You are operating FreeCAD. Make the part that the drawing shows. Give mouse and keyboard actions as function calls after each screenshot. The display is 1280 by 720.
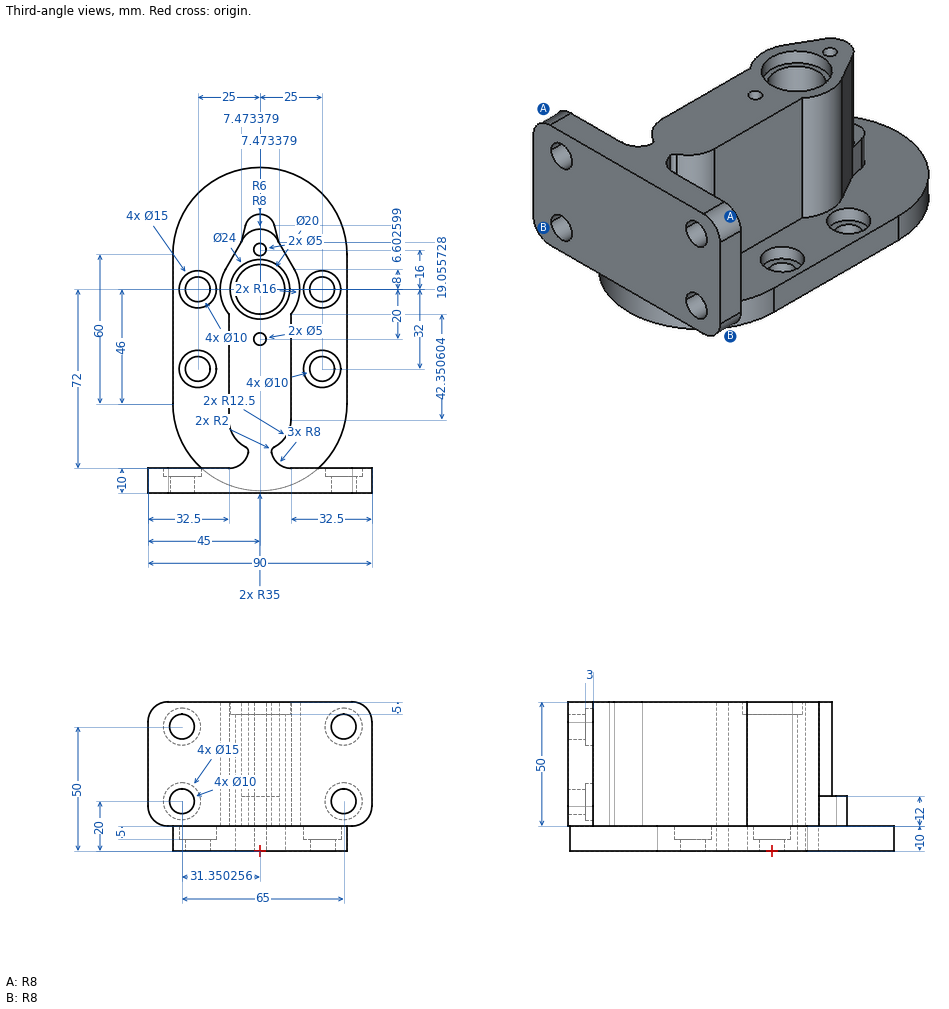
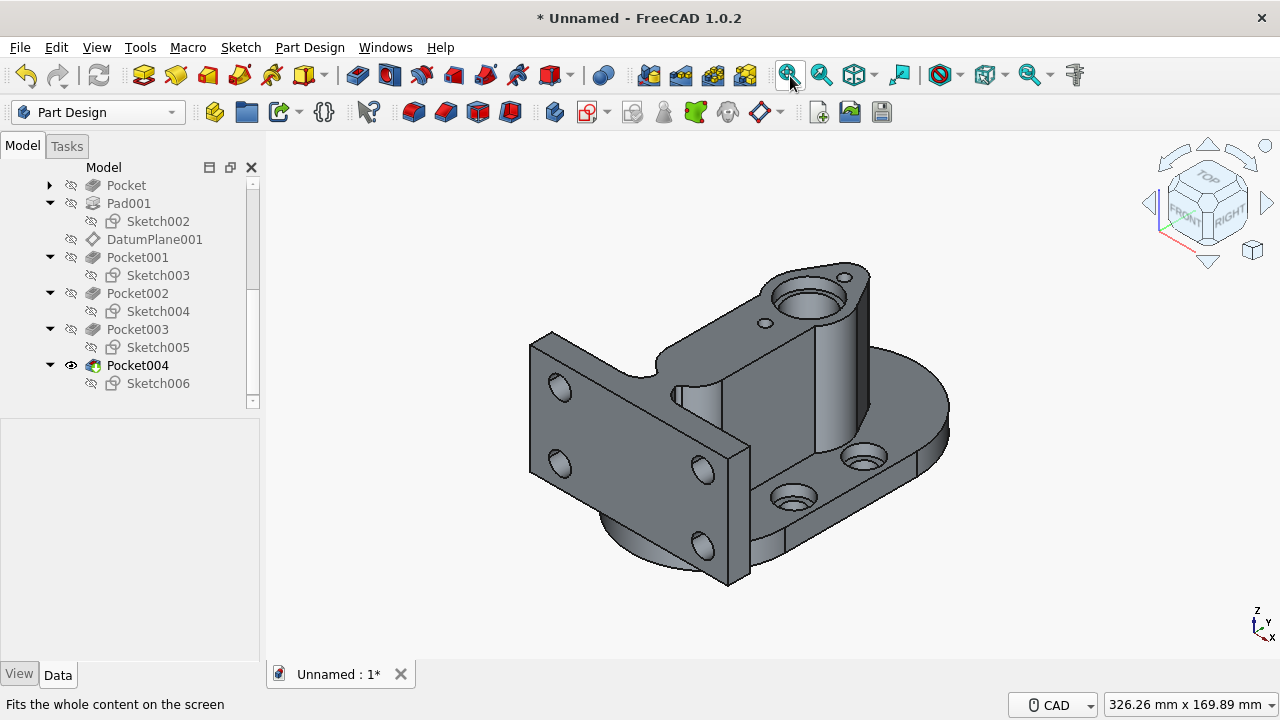
click(904, 420)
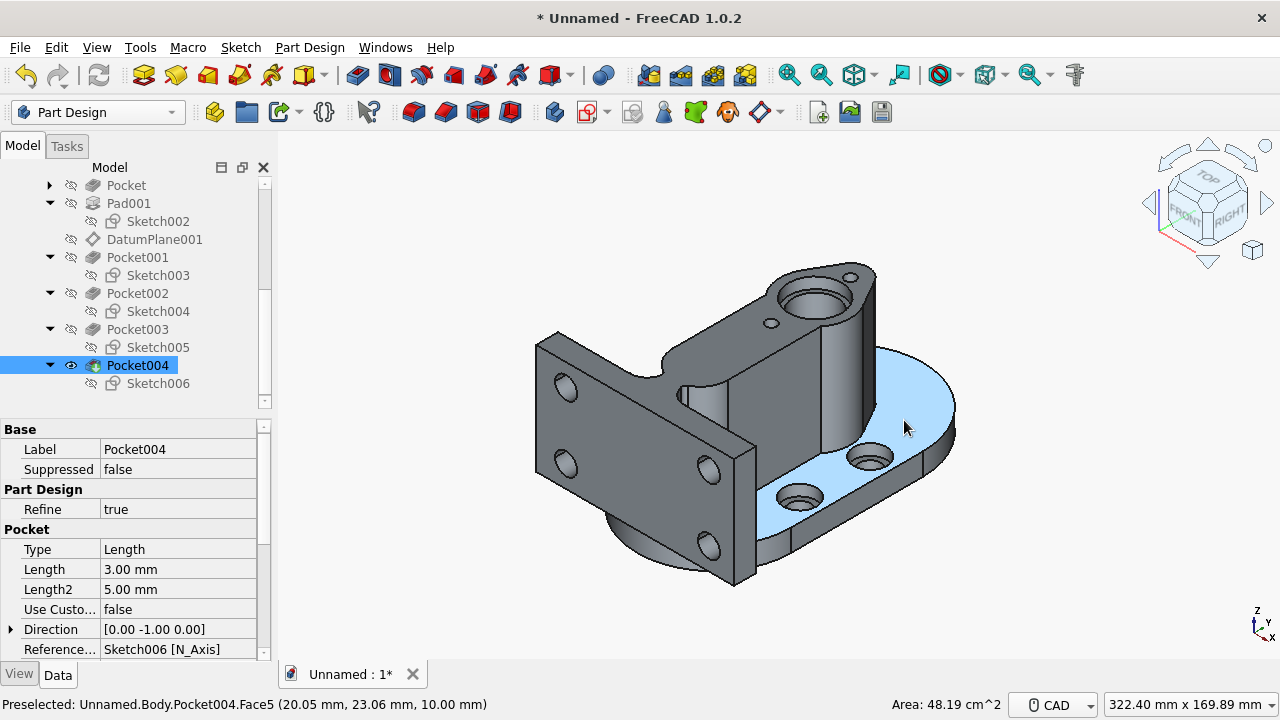
click(588, 112)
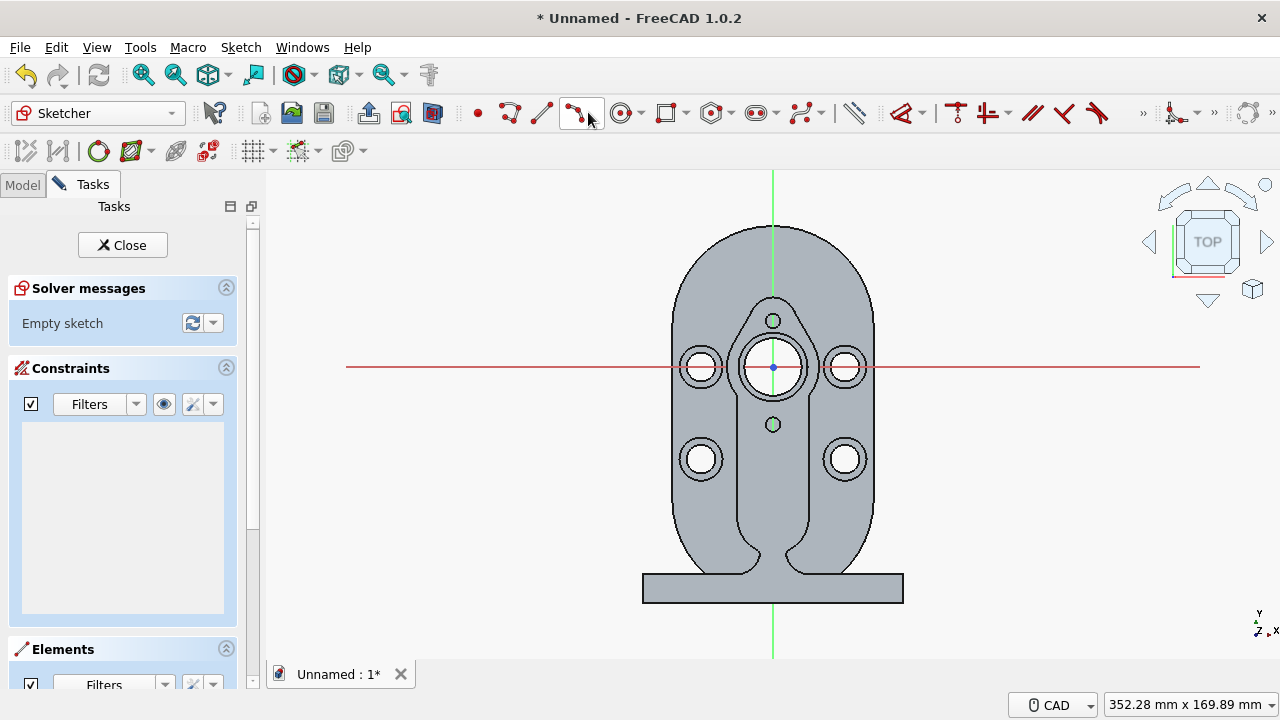
click(434, 114)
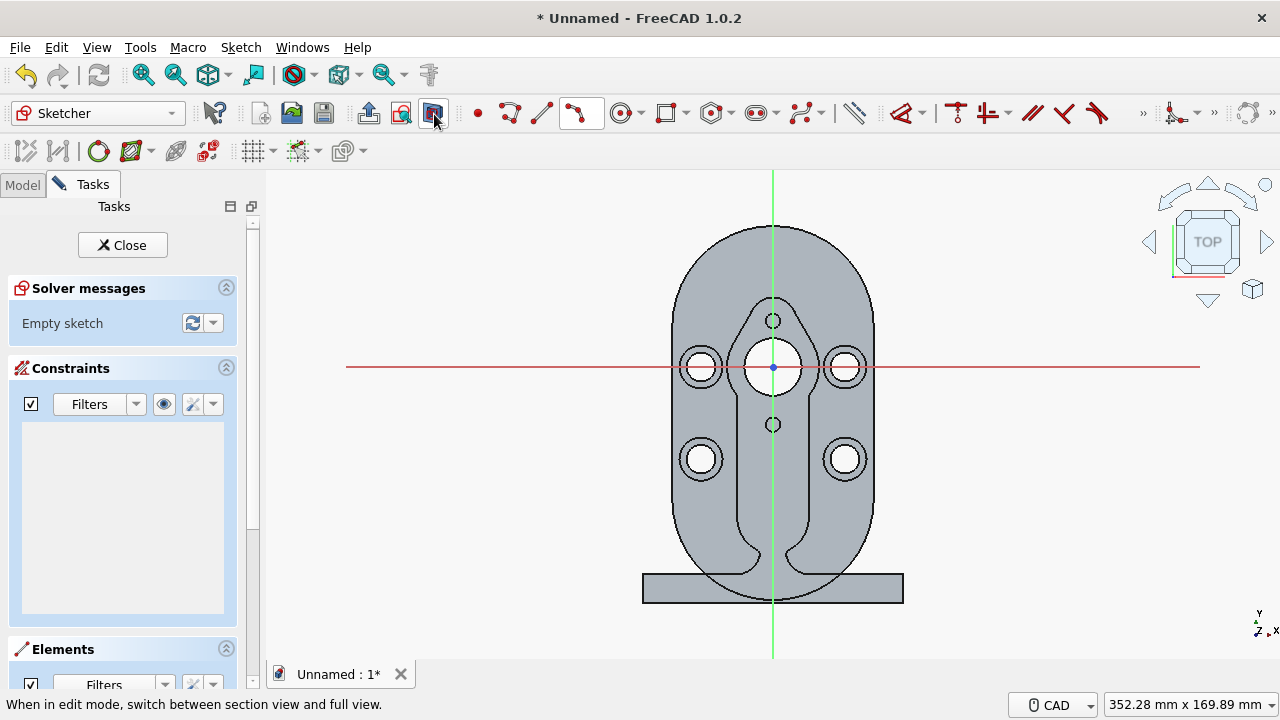
scroll(803, 284, up, 6)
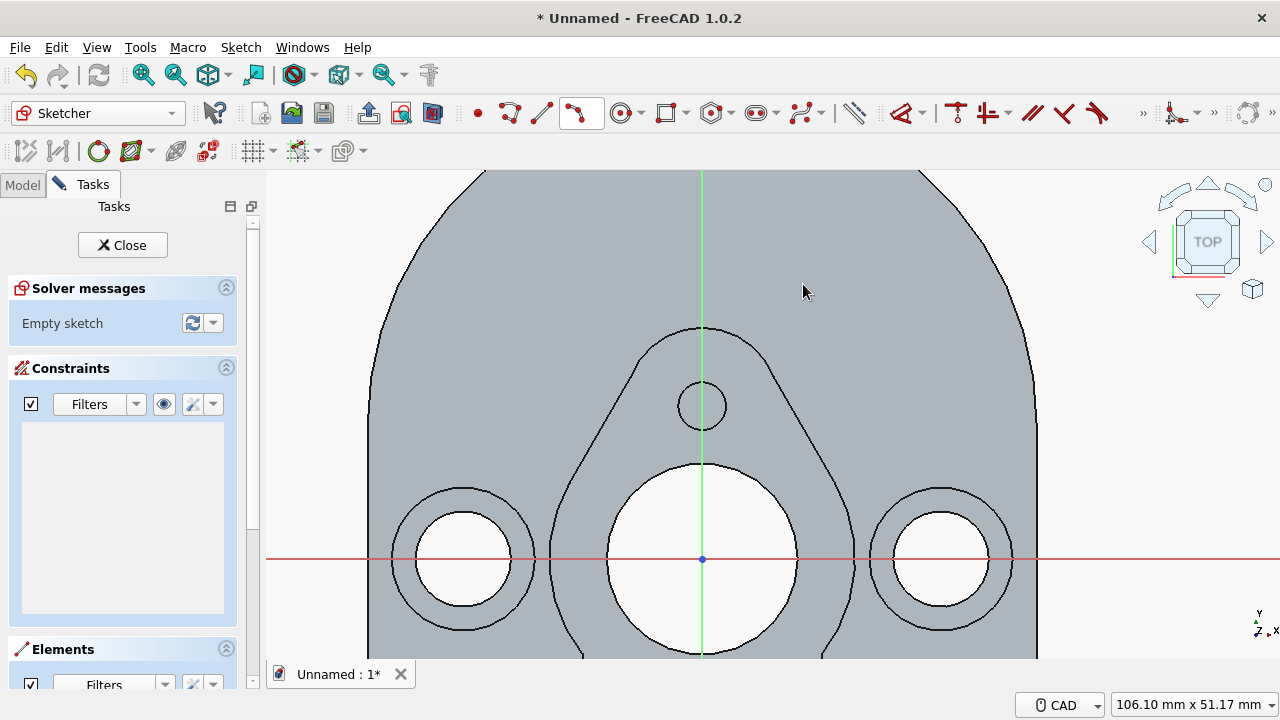
click(542, 114)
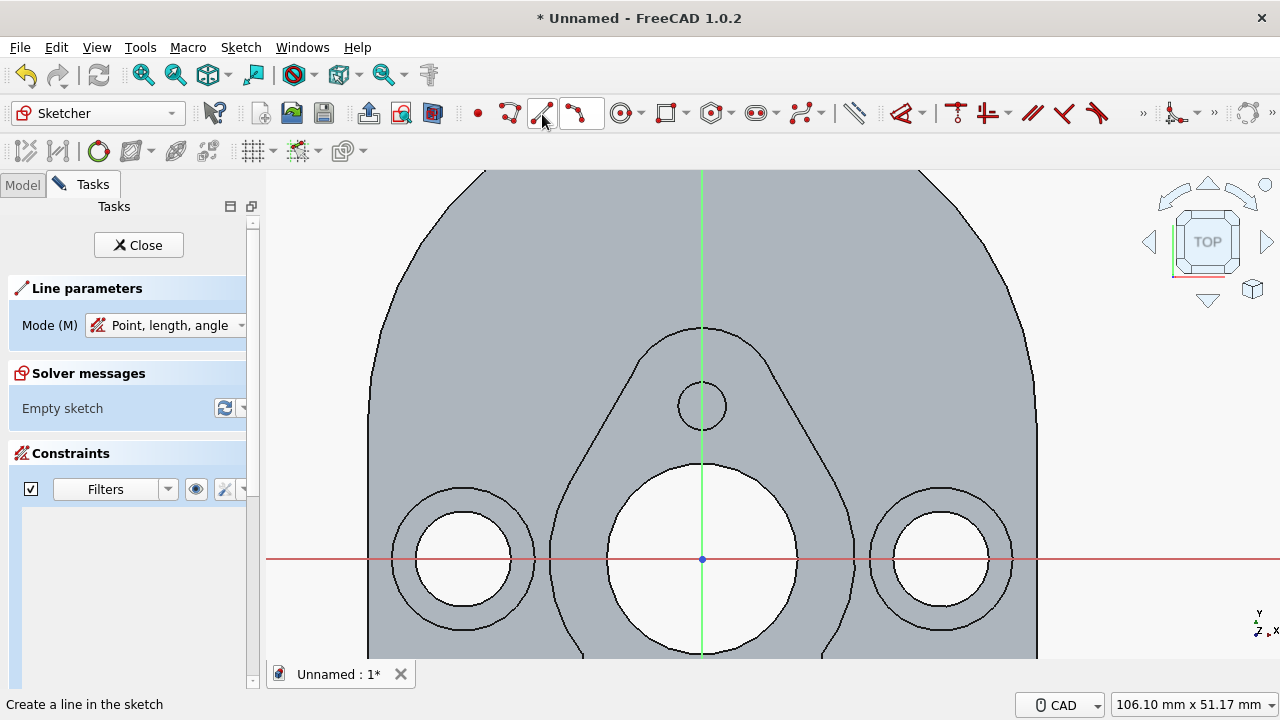
click(774, 377)
click(758, 314)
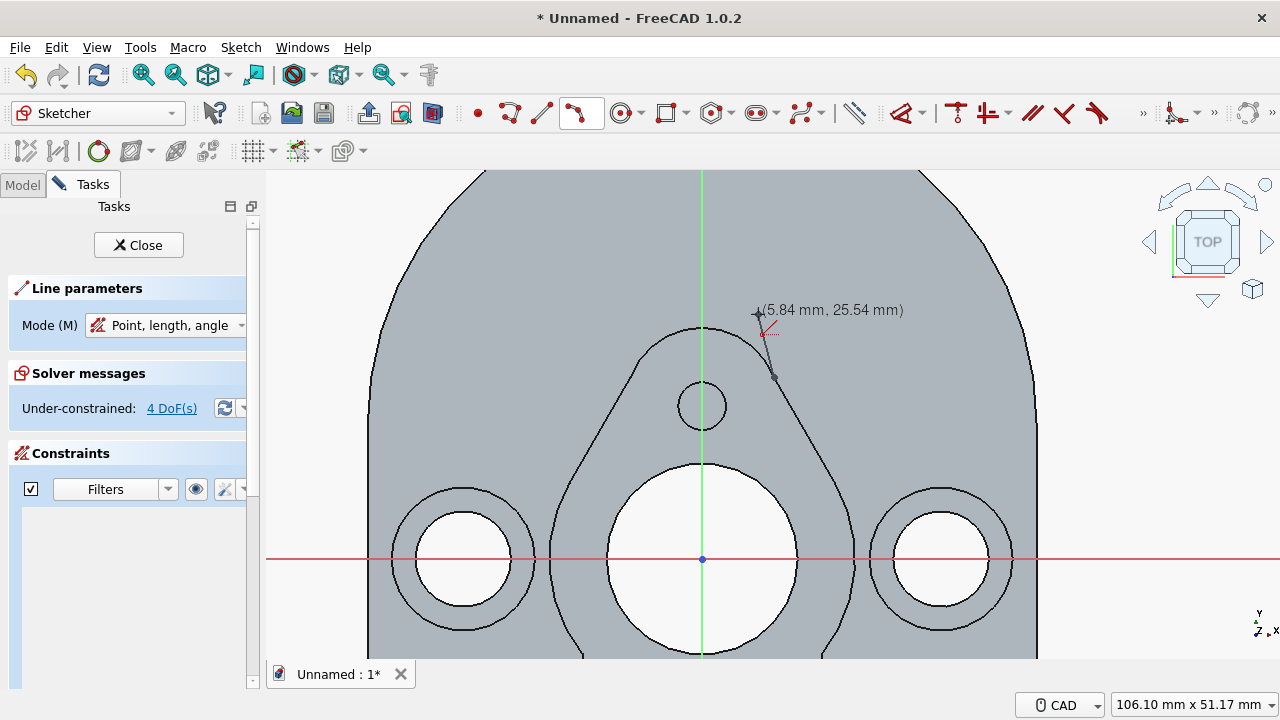
click(647, 314)
click(631, 377)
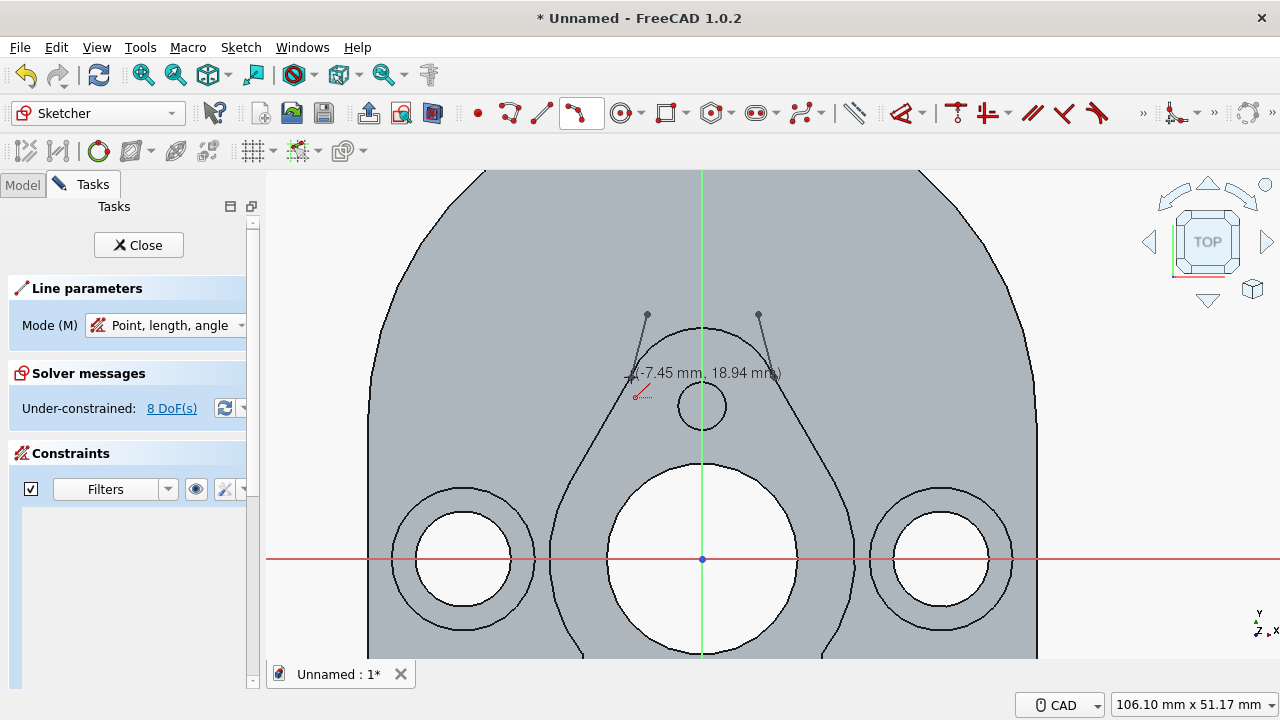
click(576, 114)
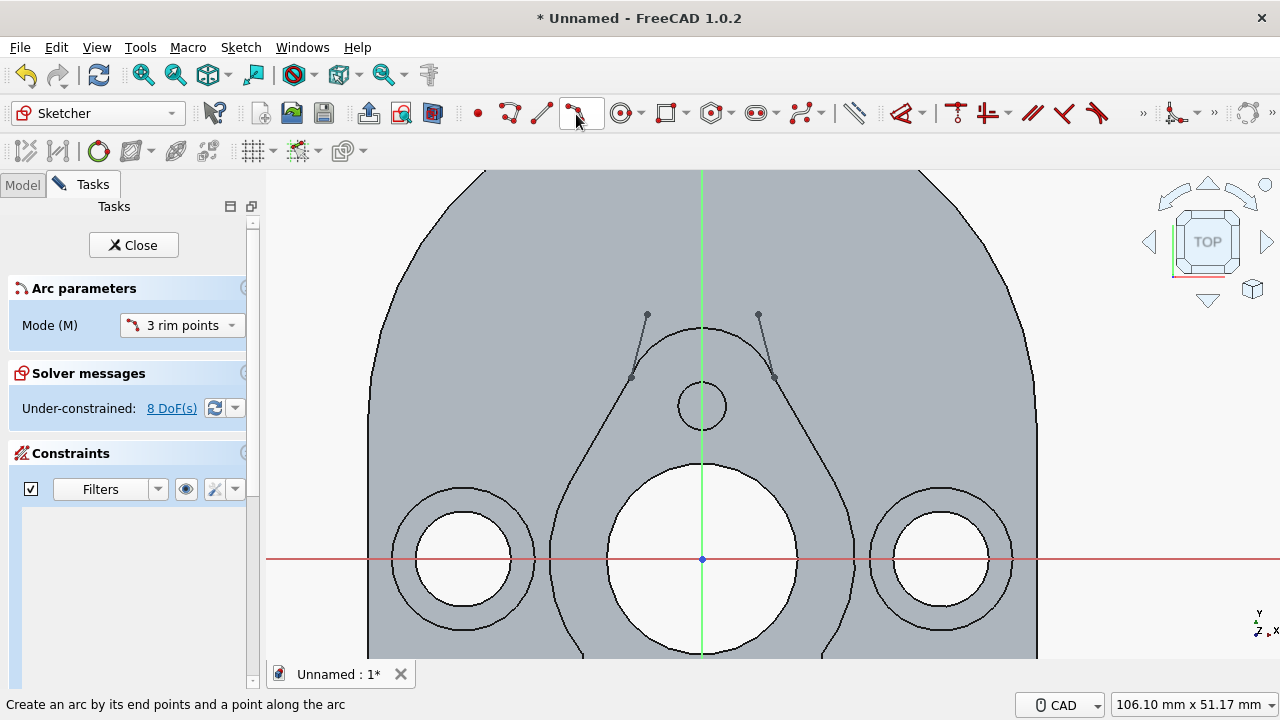
click(758, 315)
click(647, 315)
click(717, 272)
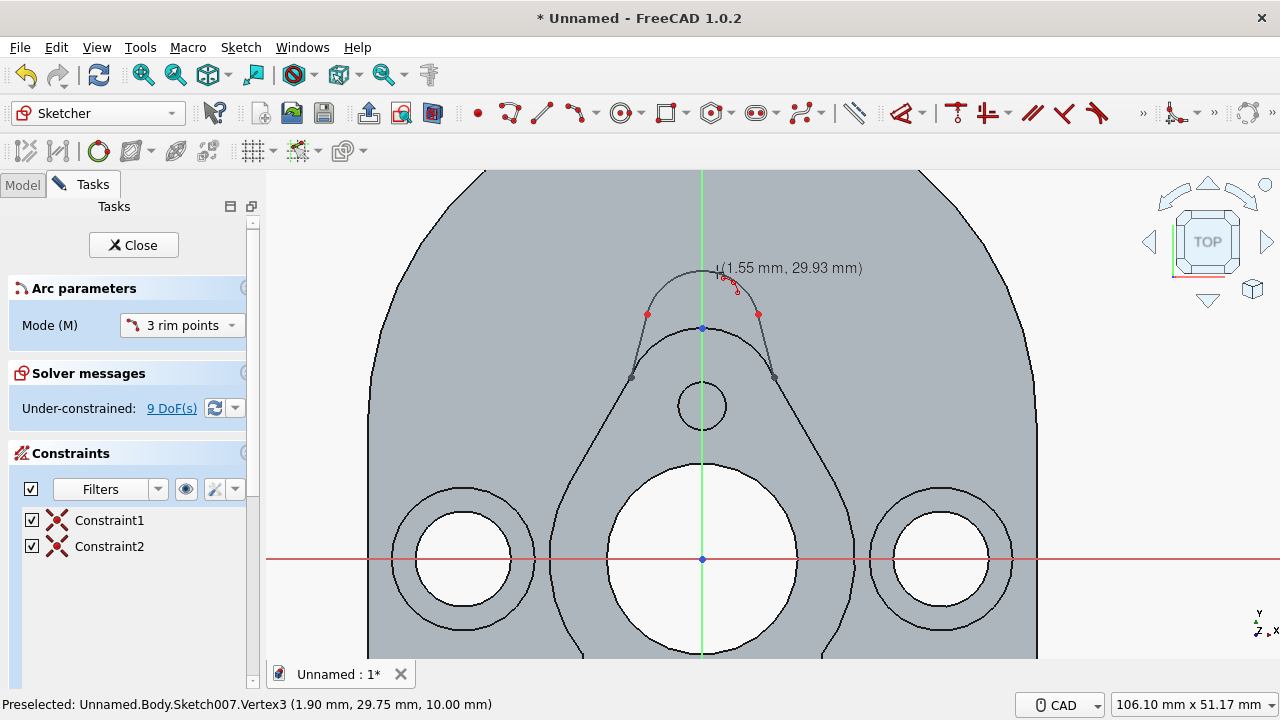
click(631, 378)
click(774, 378)
click(720, 330)
key(Escape)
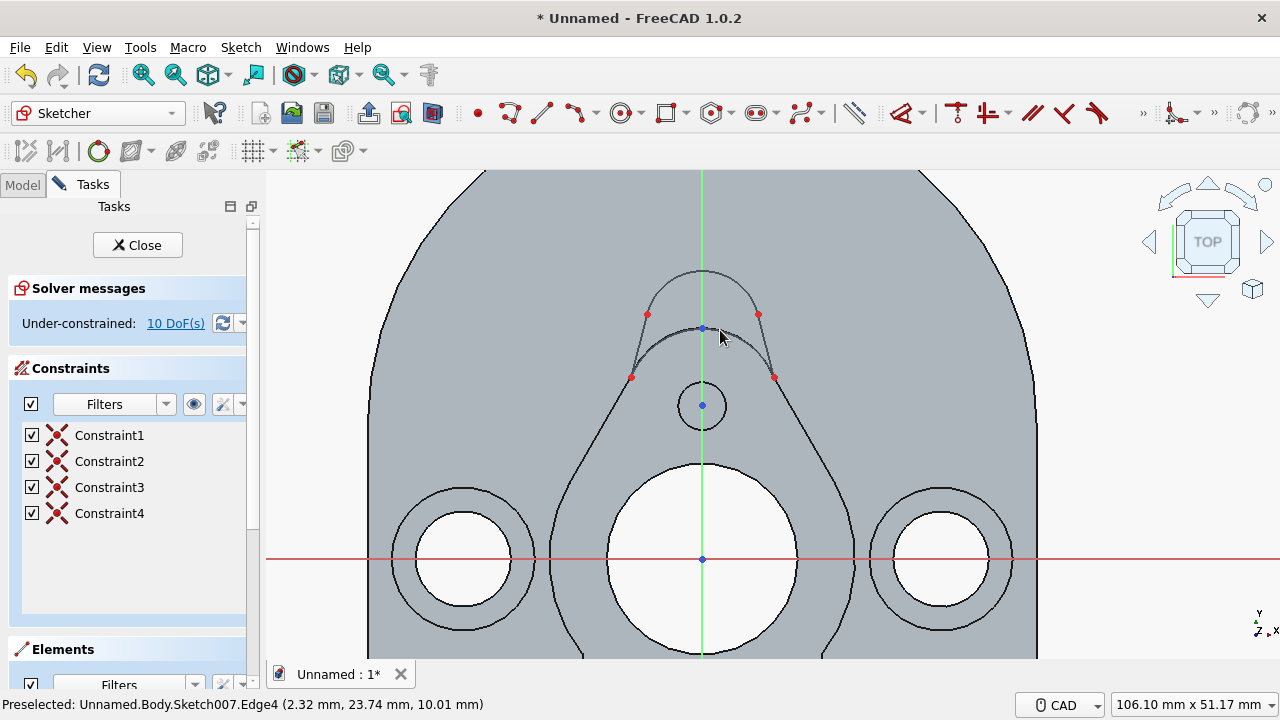
click(763, 334)